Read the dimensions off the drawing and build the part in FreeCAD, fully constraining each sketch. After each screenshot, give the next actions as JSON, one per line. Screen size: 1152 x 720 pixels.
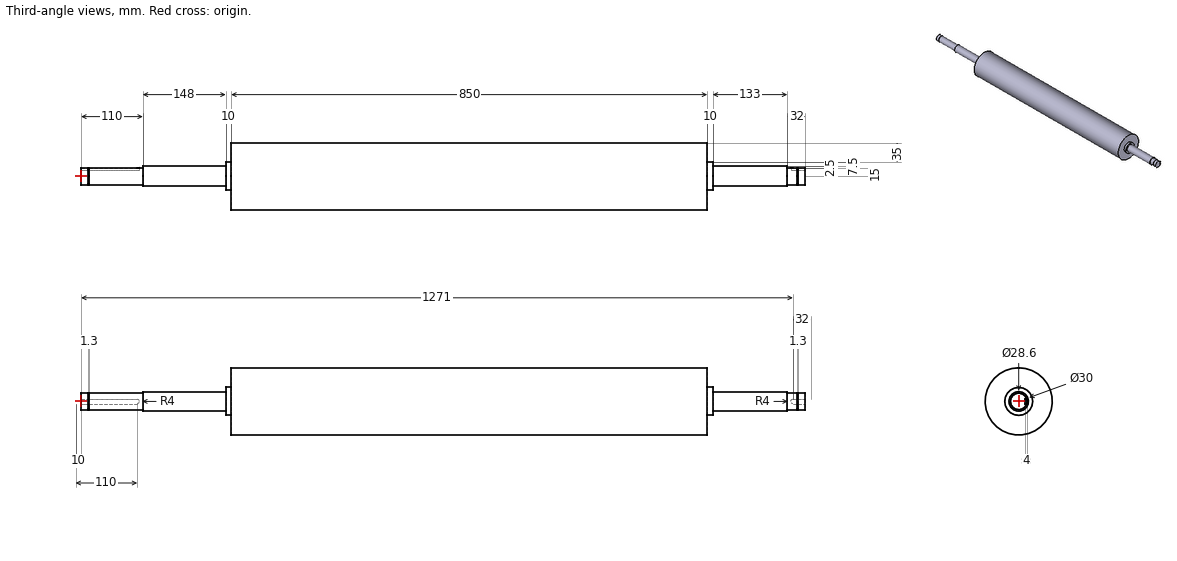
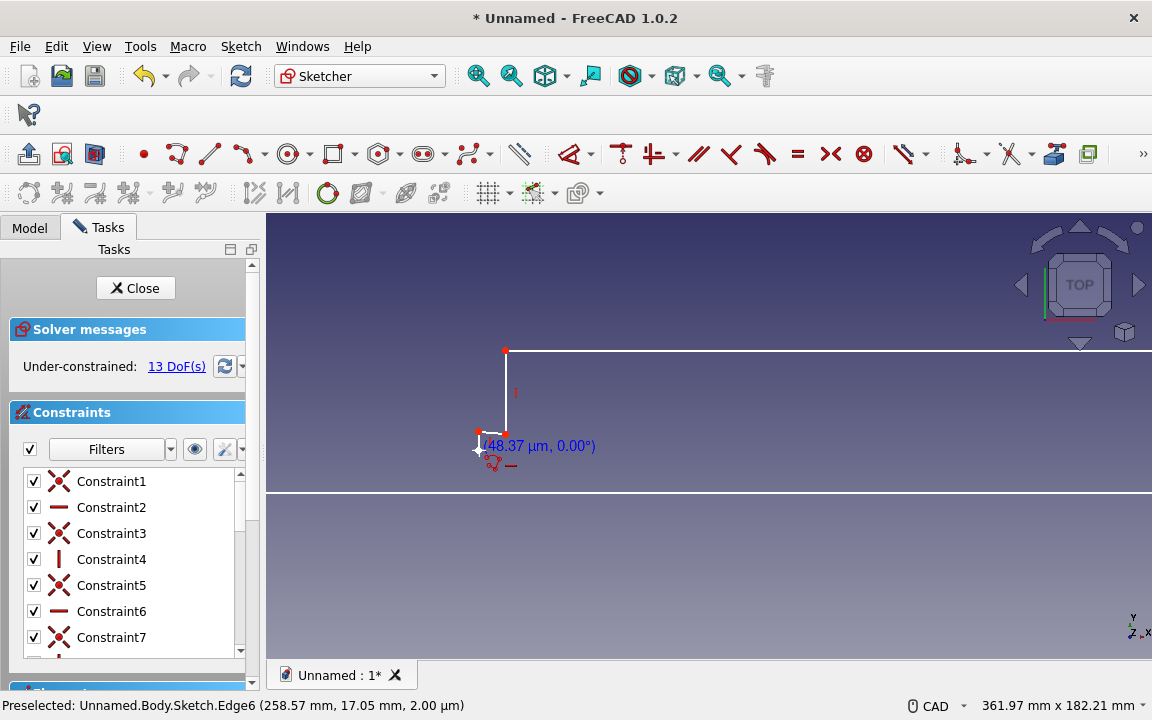
{"action": "scroll", "coordinate": [484, 439], "scroll_direction": "down", "scroll_amount": 9}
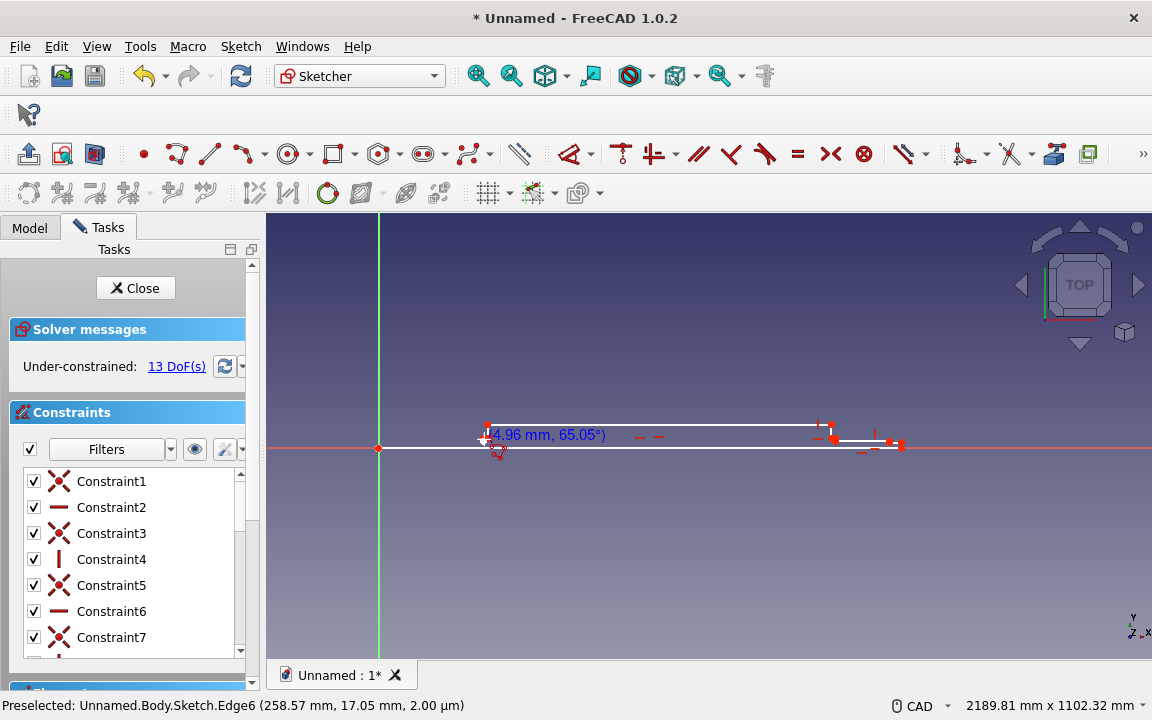
{"action": "scroll", "coordinate": [423, 441], "scroll_direction": "up", "scroll_amount": 5}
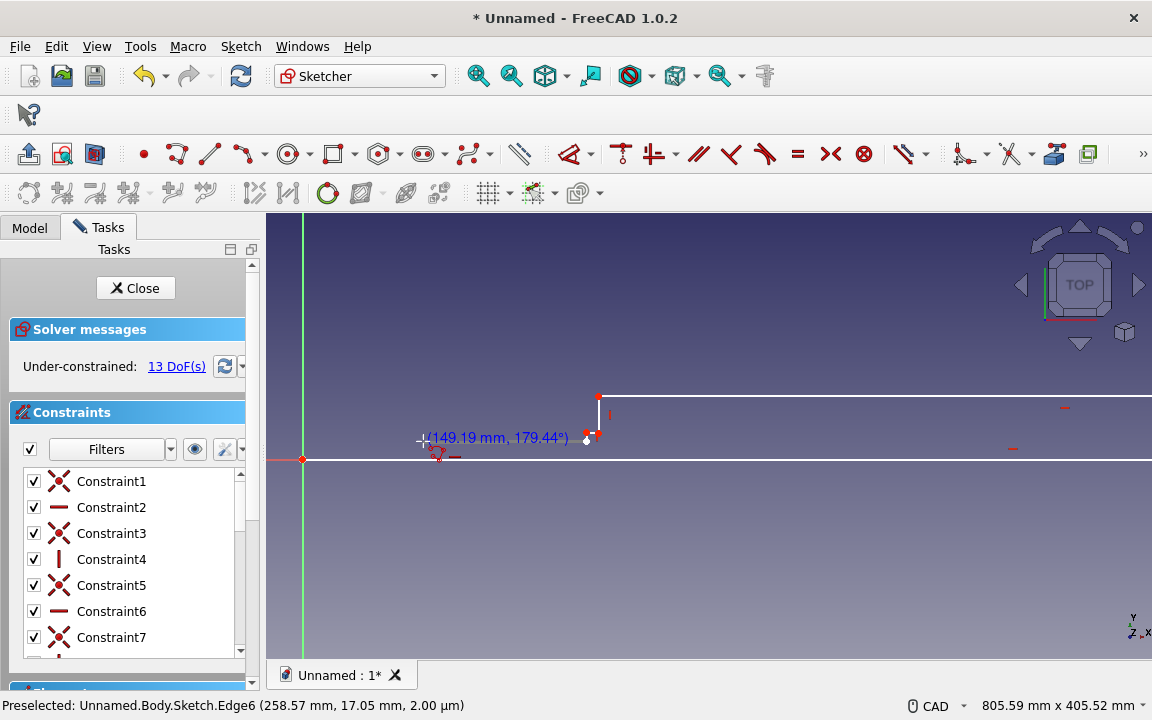
{"action": "left_click", "coordinate": [424, 441]}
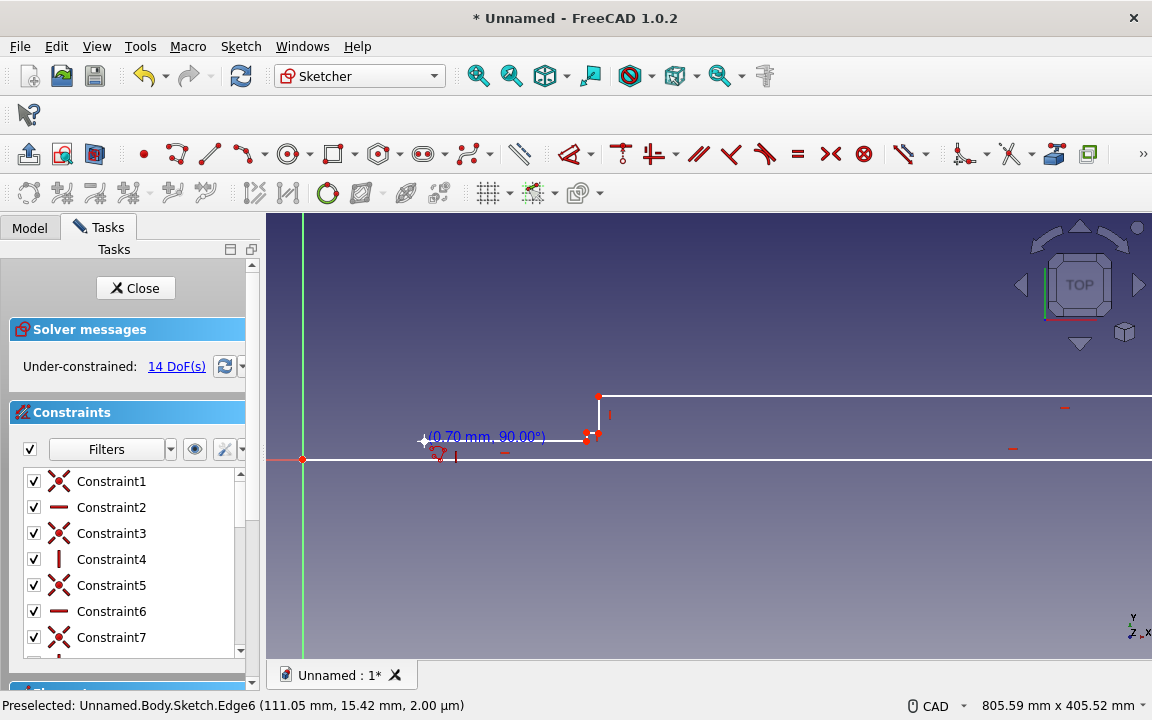
{"action": "scroll", "coordinate": [424, 443], "scroll_direction": "up", "scroll_amount": 9}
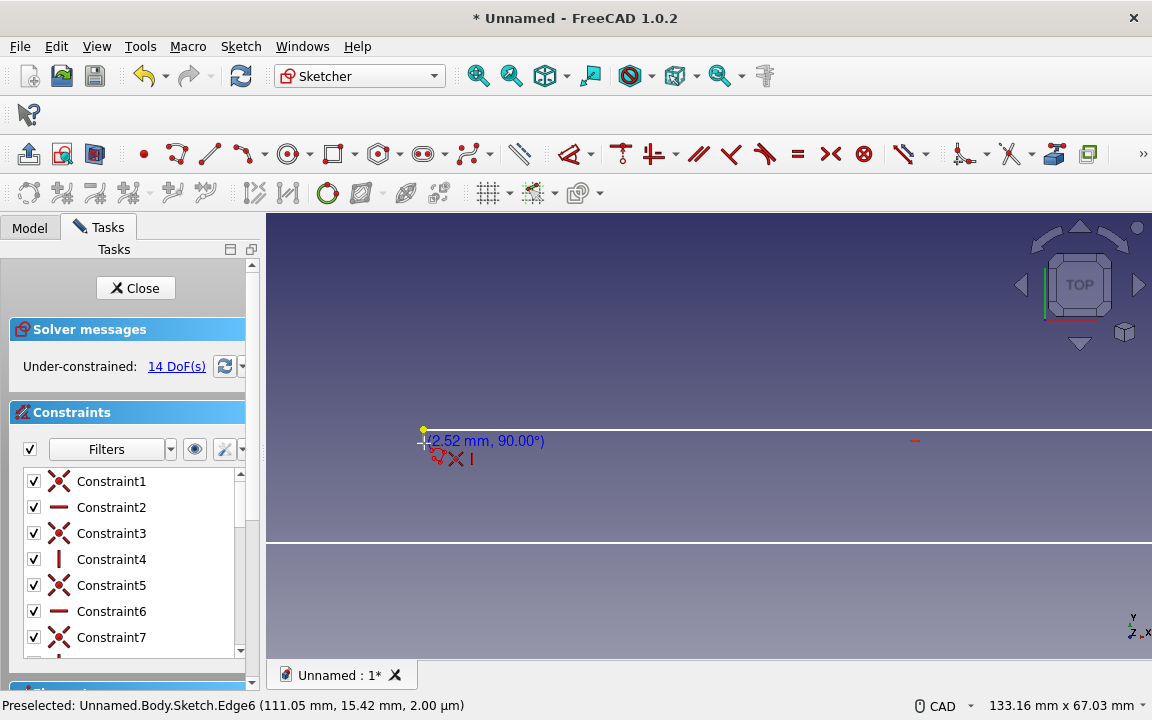
{"action": "left_click", "coordinate": [423, 443]}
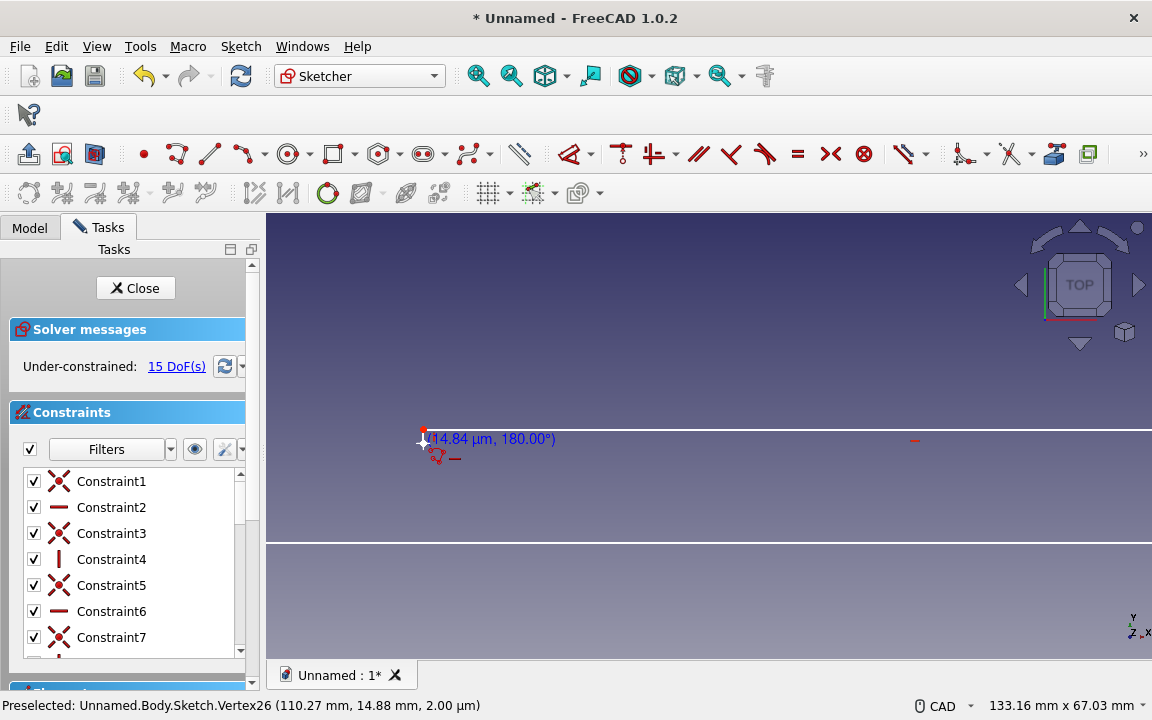
{"action": "scroll", "coordinate": [424, 442], "scroll_direction": "down", "scroll_amount": 14}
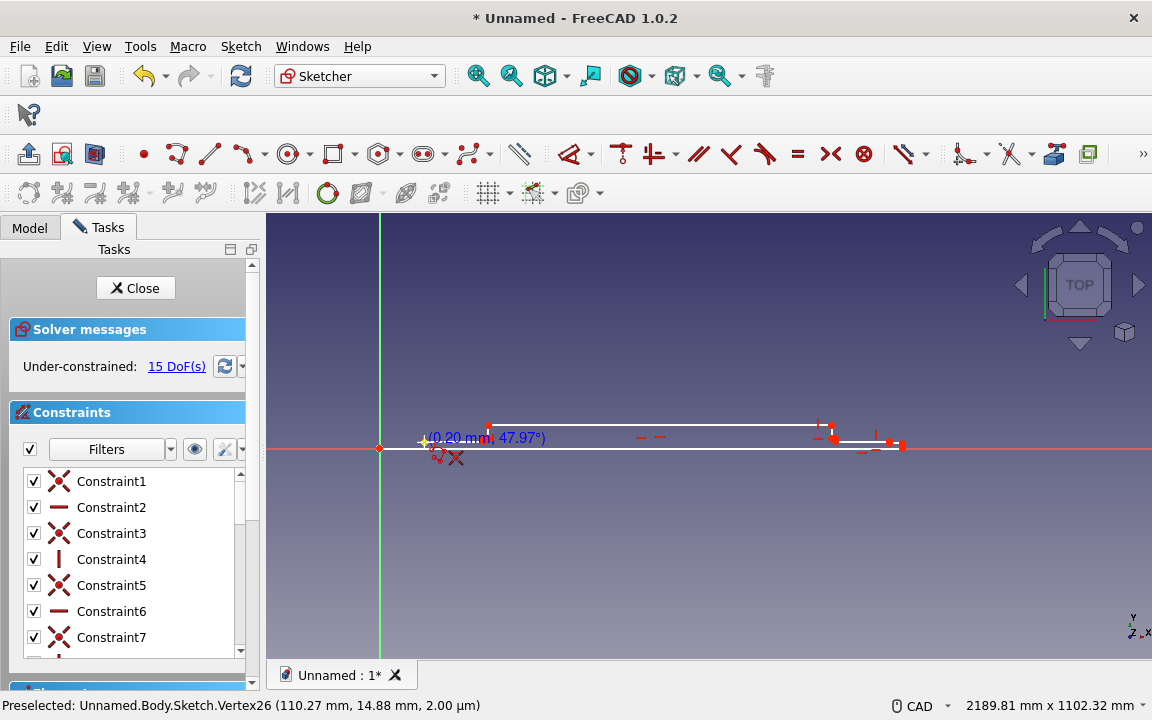
{"action": "scroll", "coordinate": [380, 443], "scroll_direction": "up", "scroll_amount": 5}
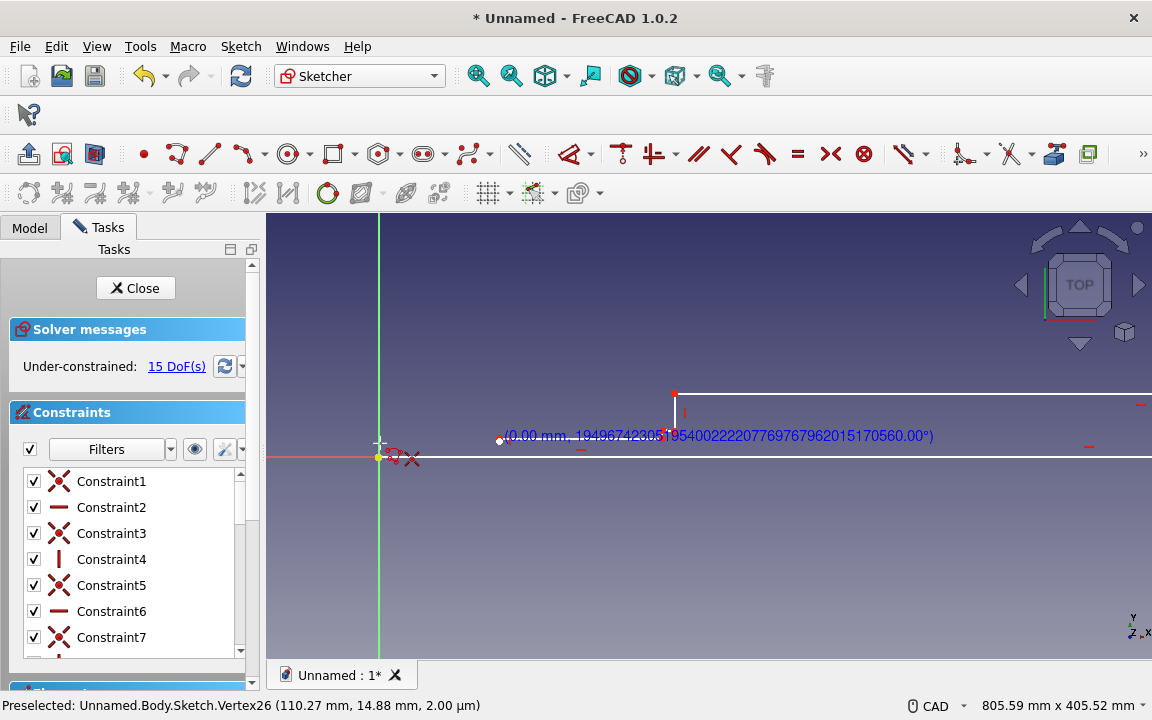
{"action": "left_click", "coordinate": [388, 441]}
{"action": "left_click", "coordinate": [379, 457]}
{"action": "key", "text": "Escape"}
{"action": "key", "text": "Escape"}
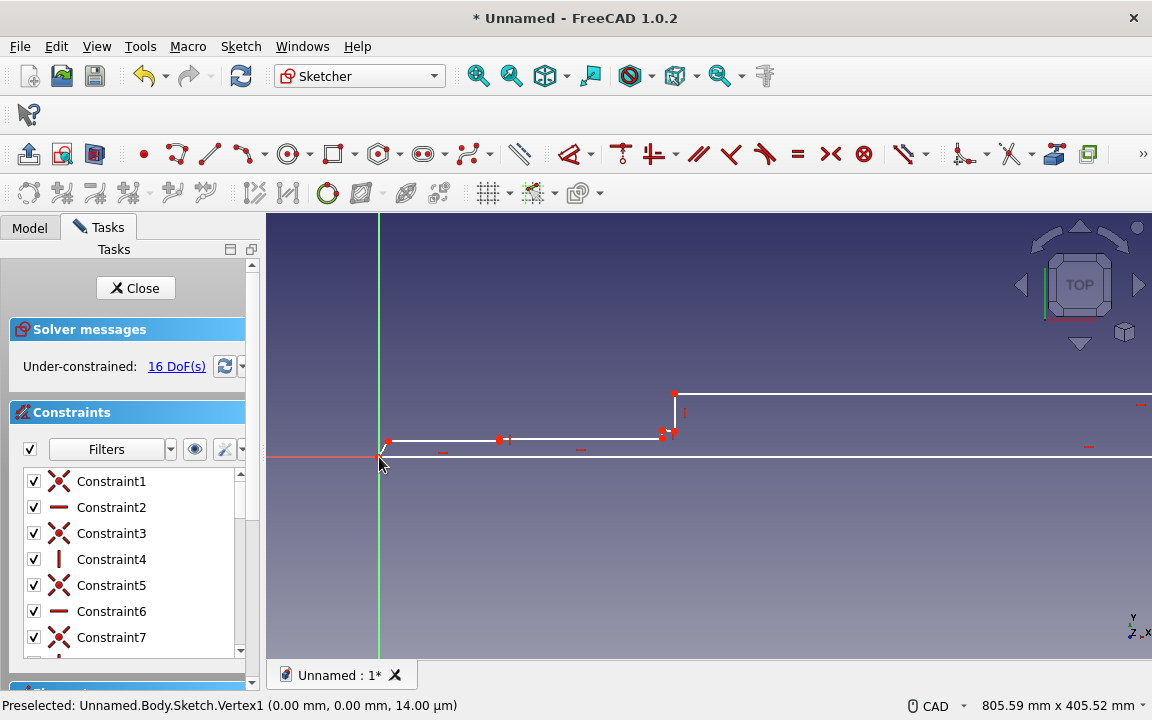
{"action": "scroll", "coordinate": [669, 431], "scroll_direction": "up", "scroll_amount": 5}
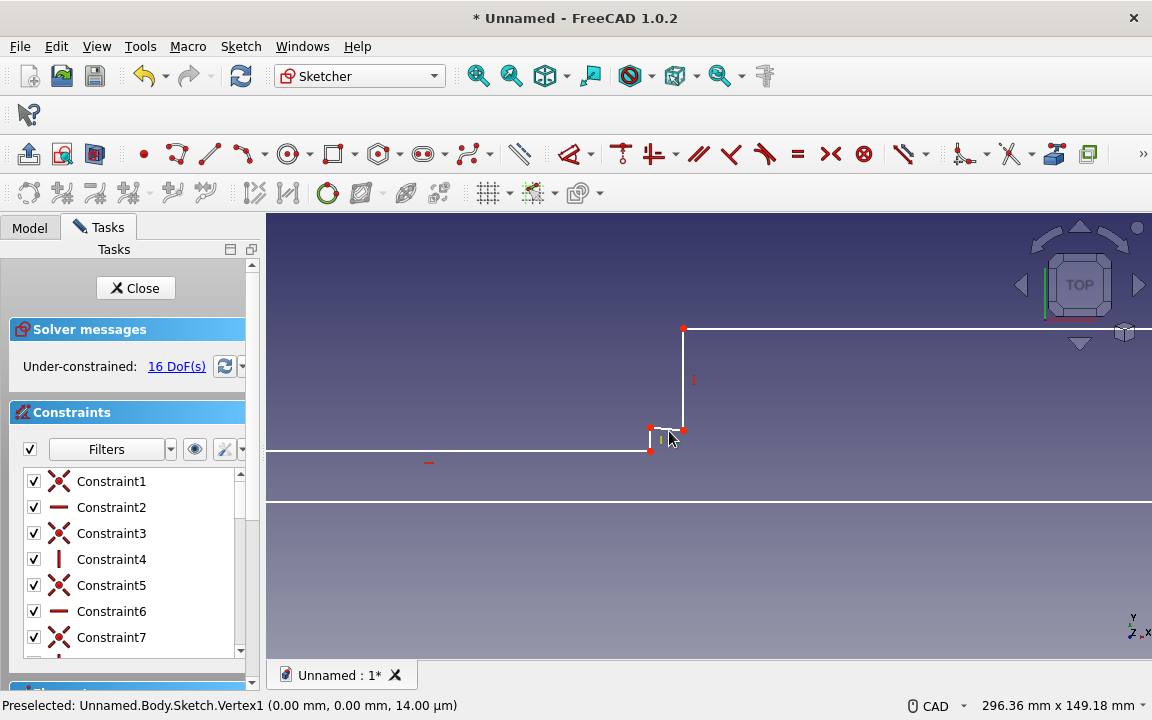
{"action": "left_click", "coordinate": [667, 429]}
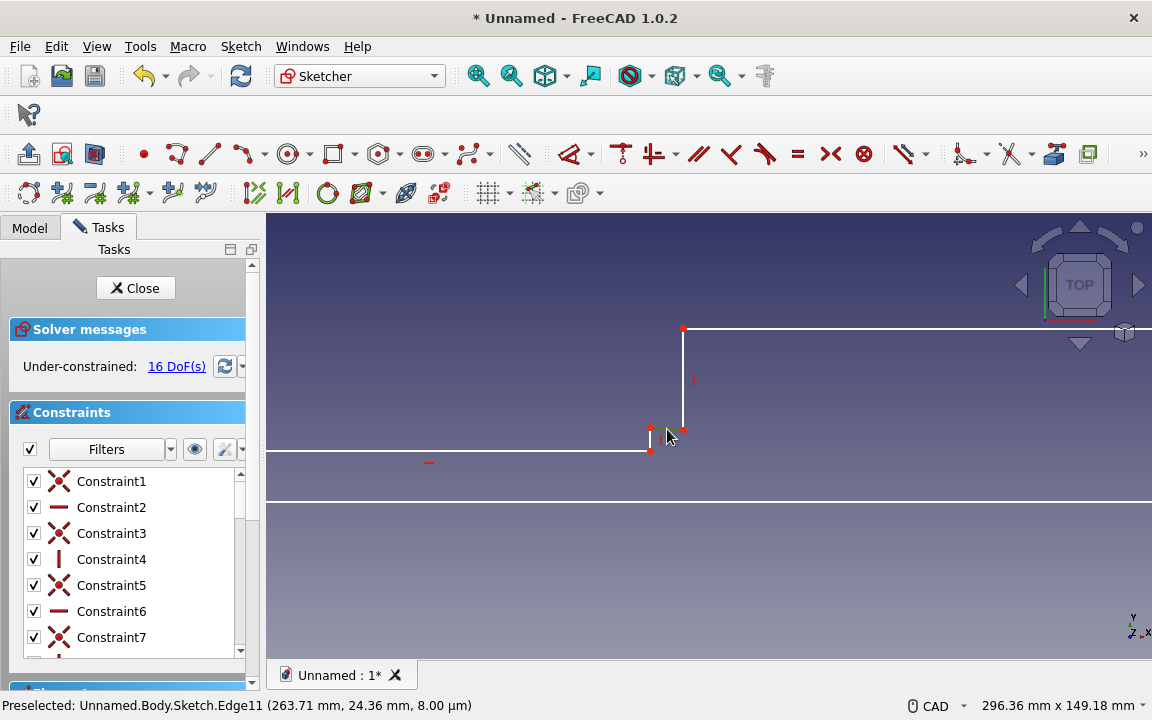
{"action": "key", "text": "h"}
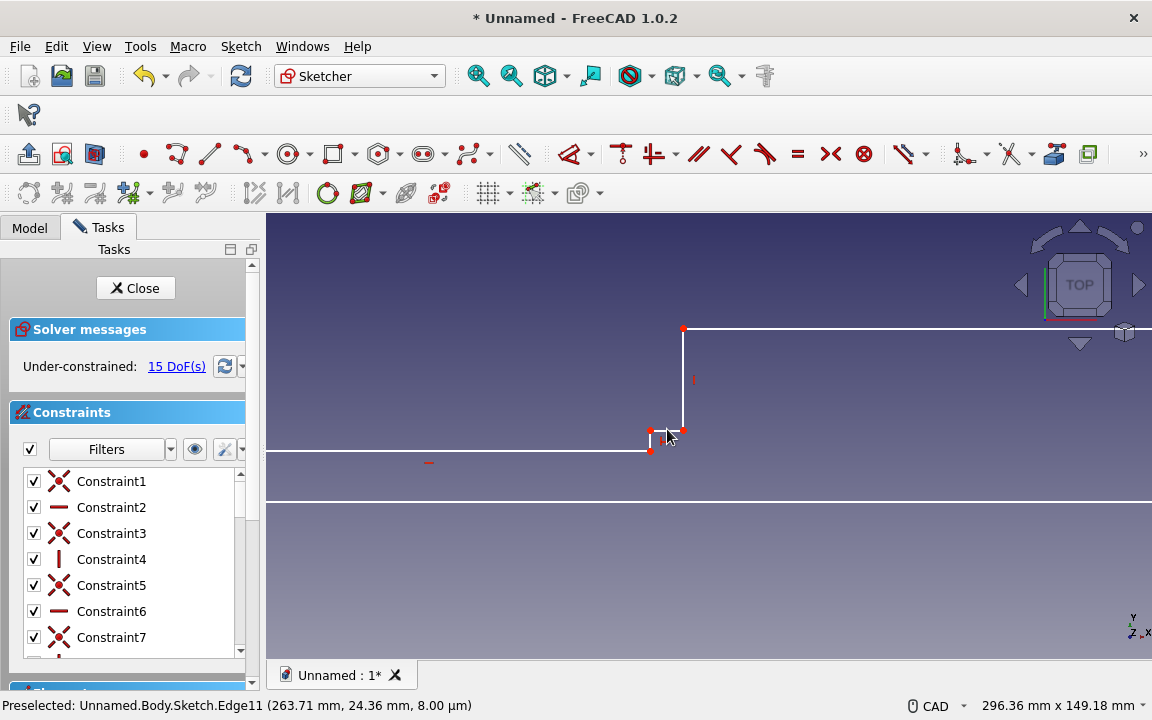
{"action": "scroll", "coordinate": [457, 440], "scroll_direction": "down", "scroll_amount": 10}